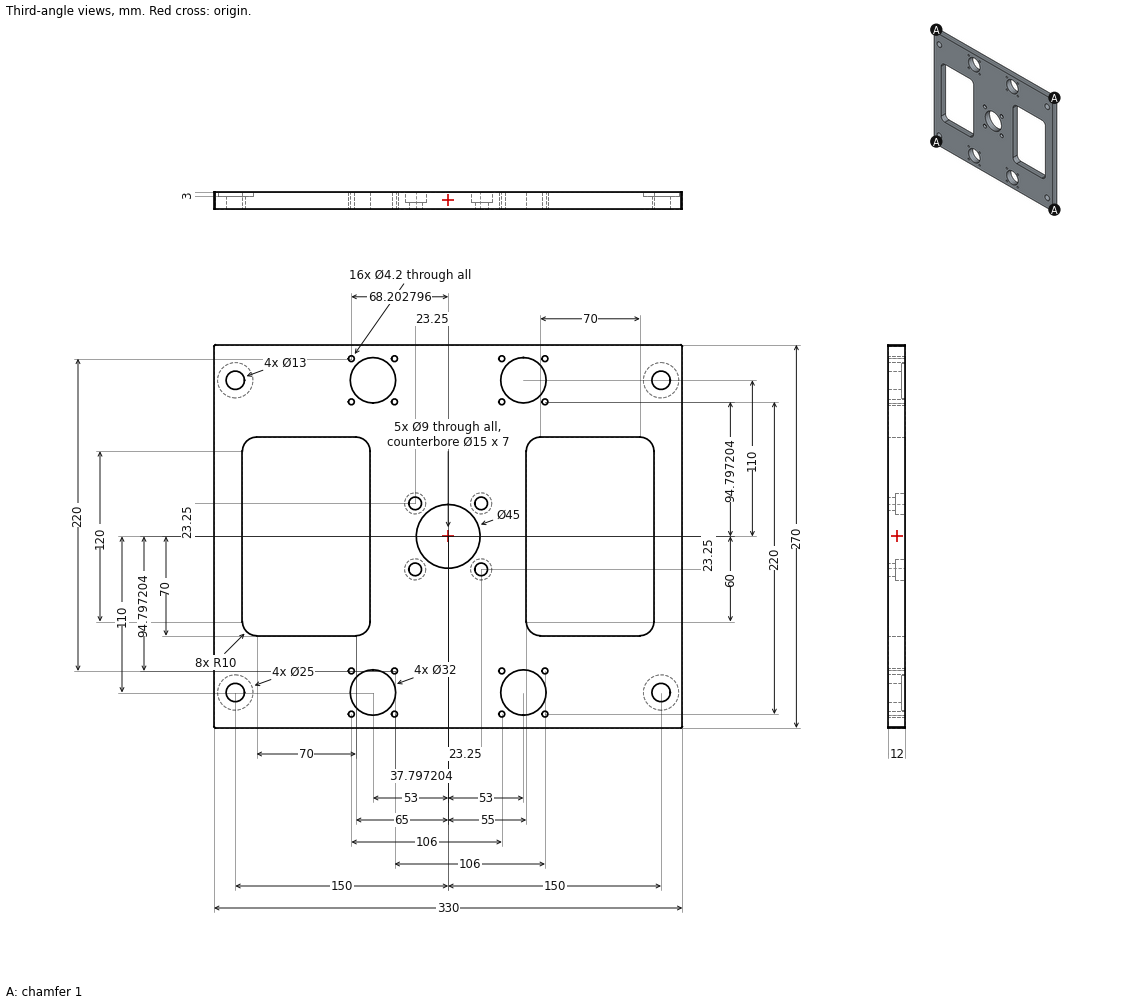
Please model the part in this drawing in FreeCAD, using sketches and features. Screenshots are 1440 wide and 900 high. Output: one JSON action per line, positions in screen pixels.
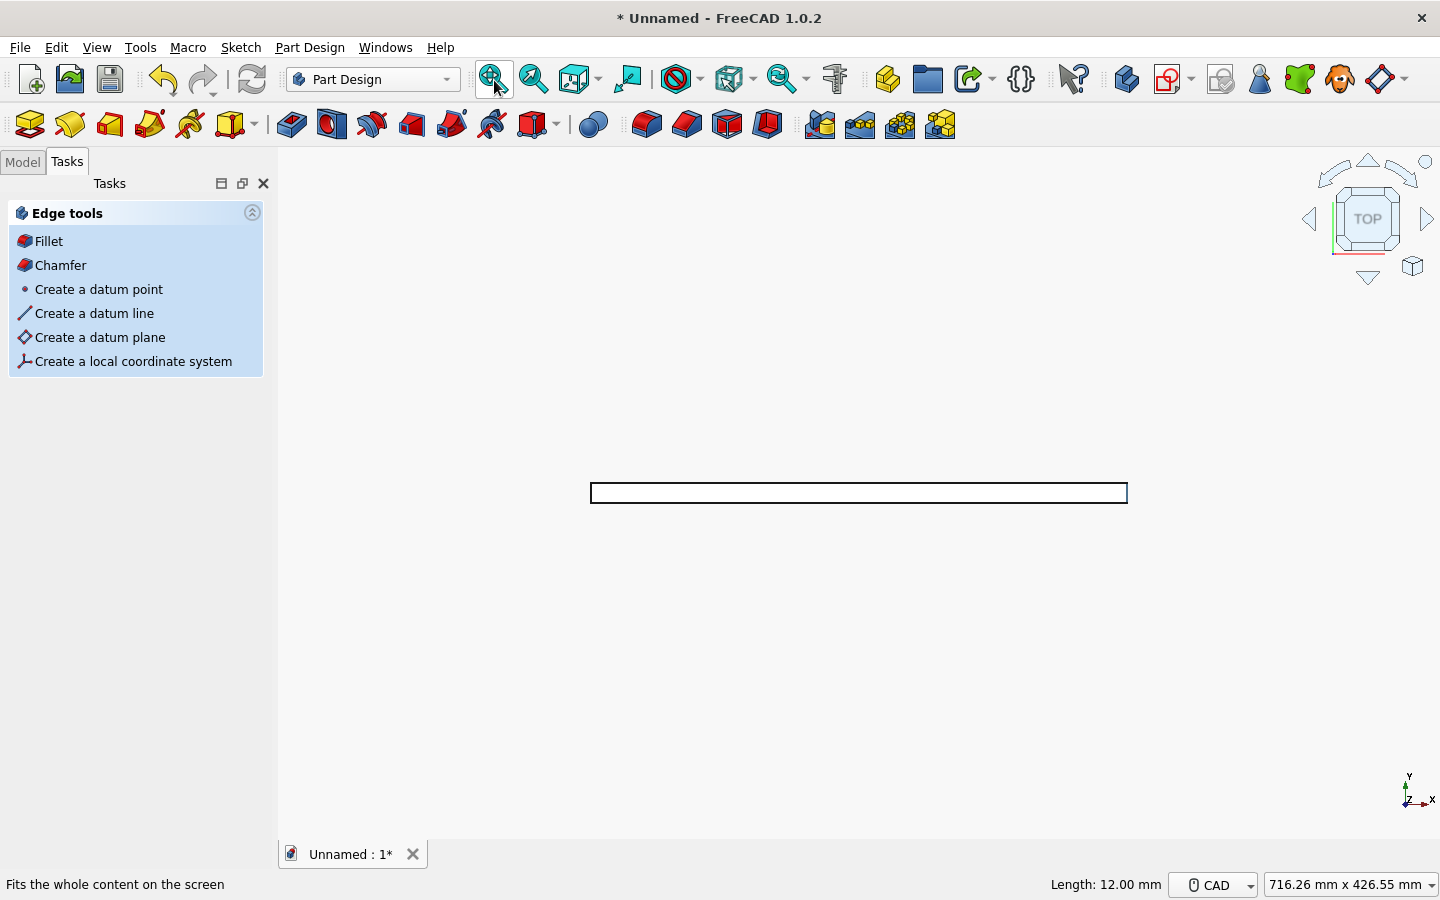
{"action": "left_click", "coordinate": [591, 492], "text": "ctrl"}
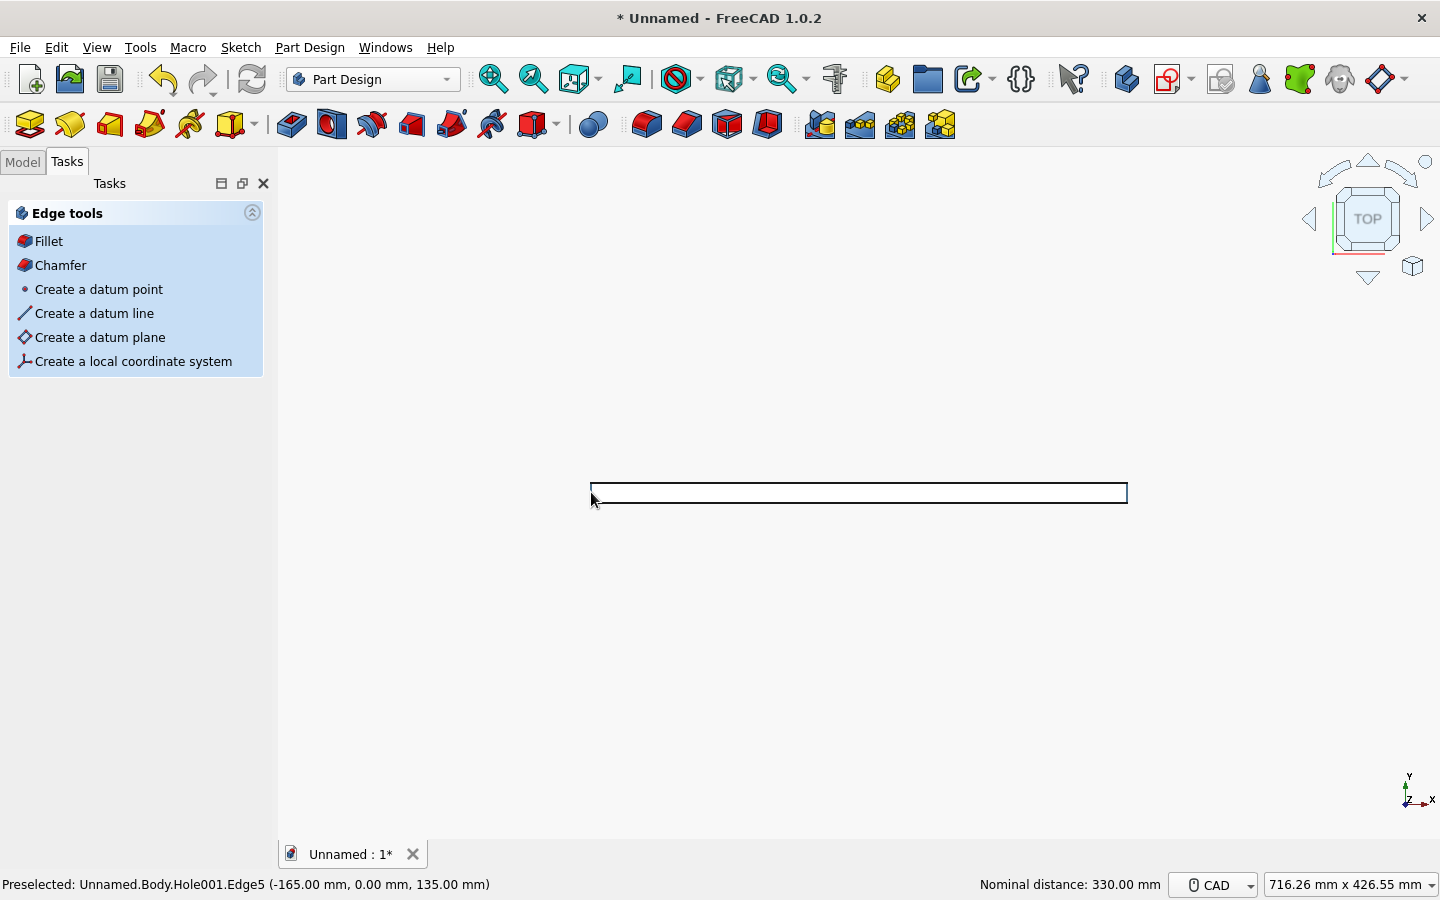
{"action": "scroll", "coordinate": [591, 492], "scroll_direction": "up", "scroll_amount": 4}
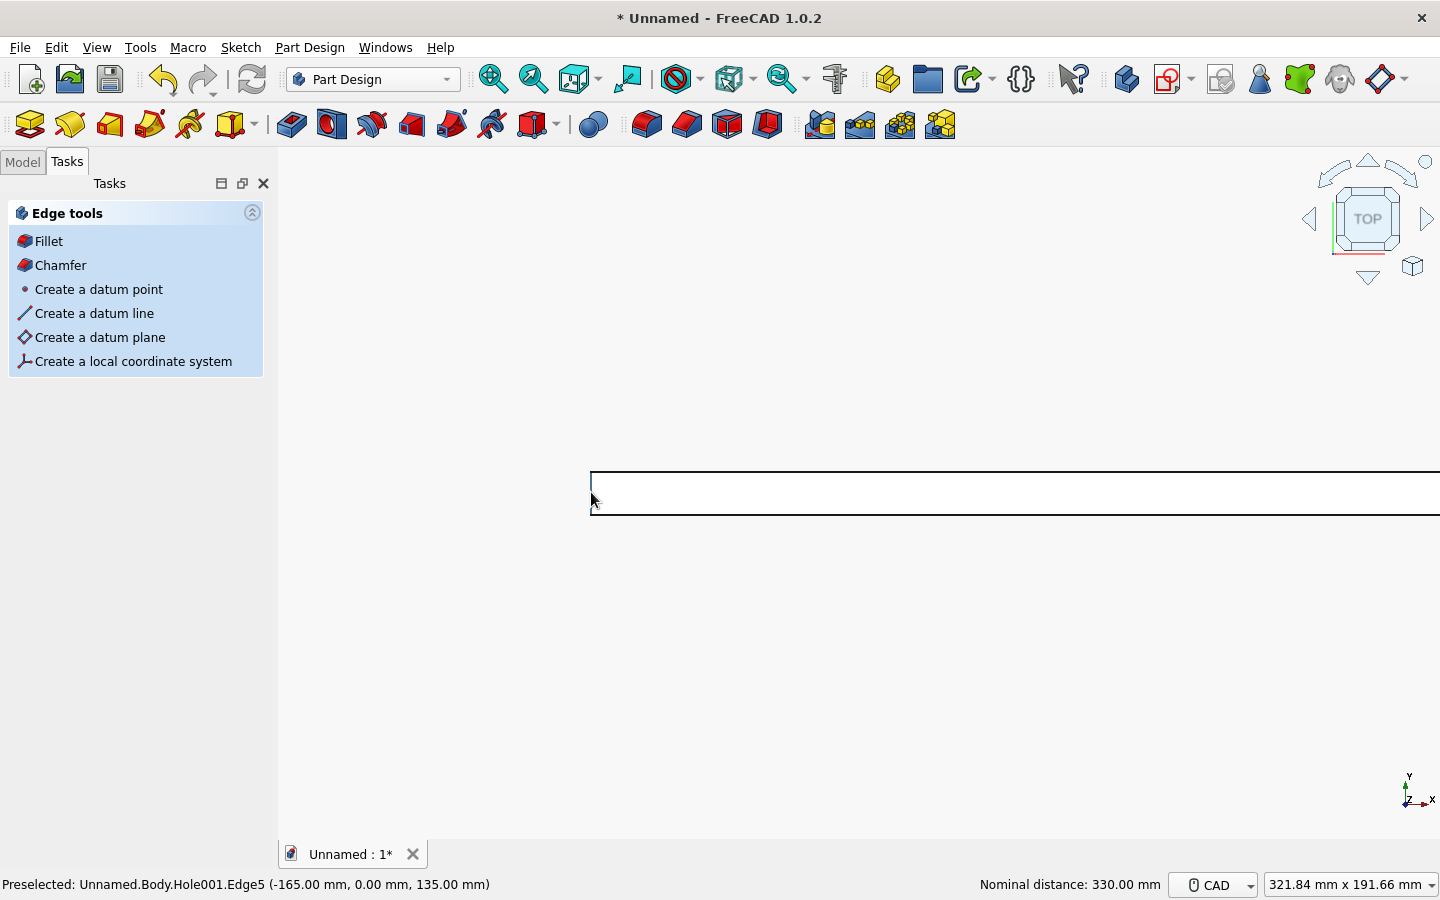
{"action": "left_click", "coordinate": [494, 80]}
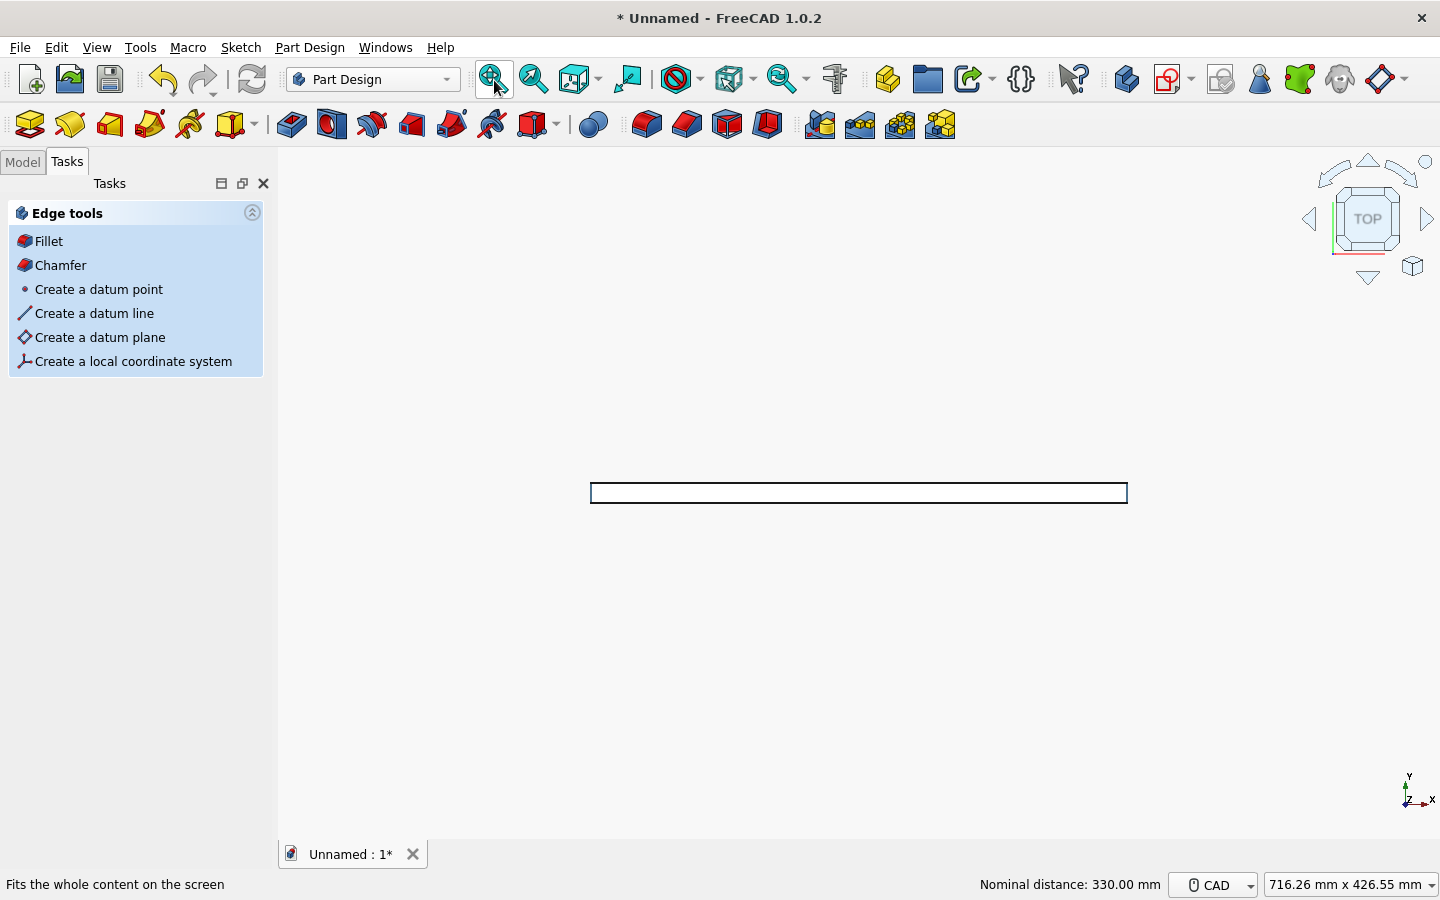
{"action": "key", "text": "1"}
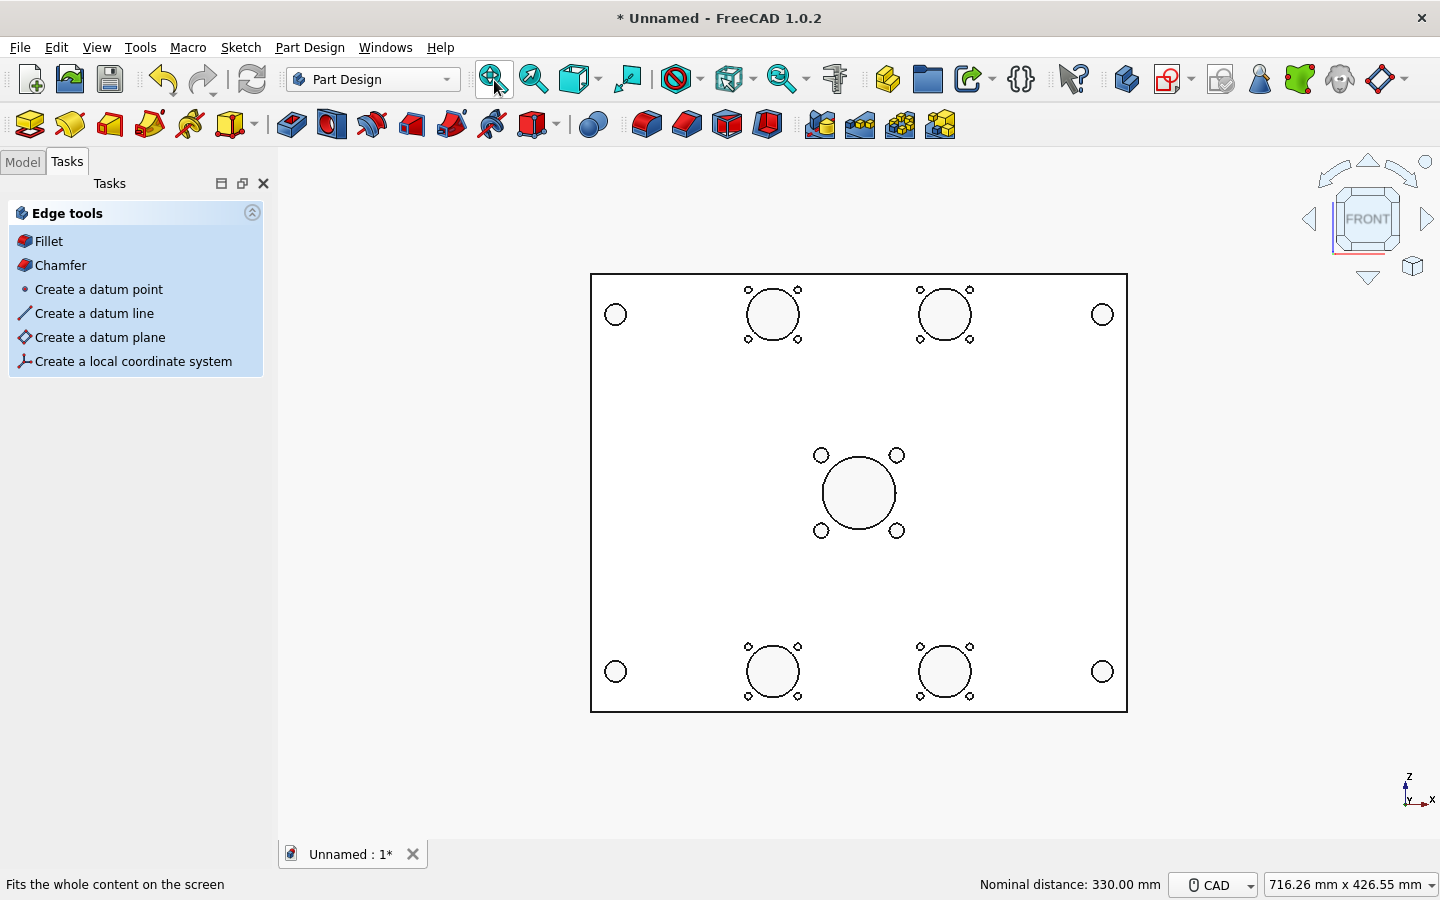
{"action": "scroll", "coordinate": [591, 711], "scroll_direction": "up", "scroll_amount": 4}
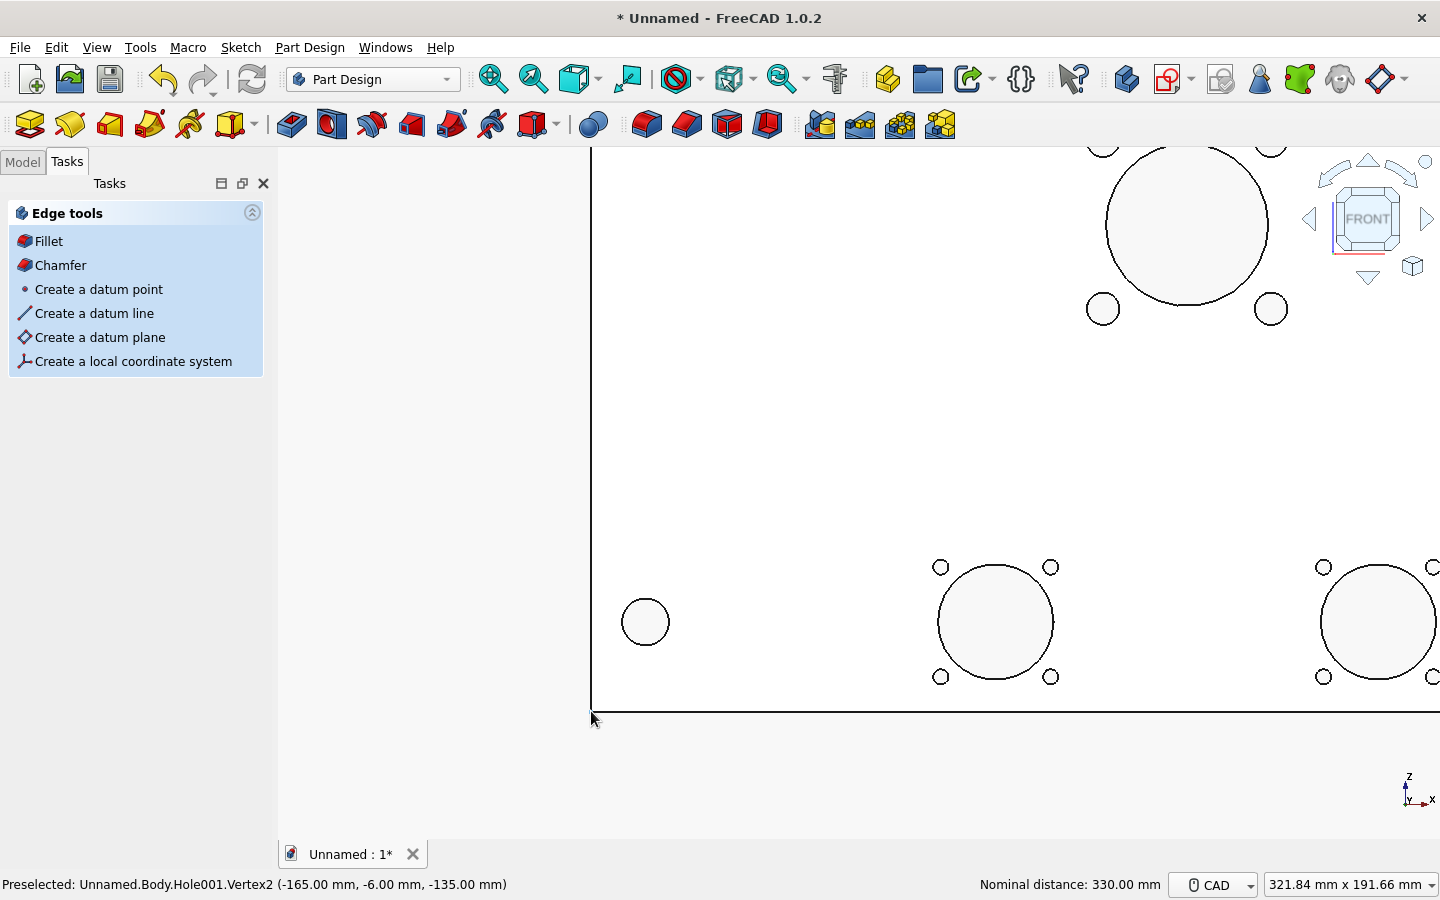
{"action": "left_click", "coordinate": [494, 80]}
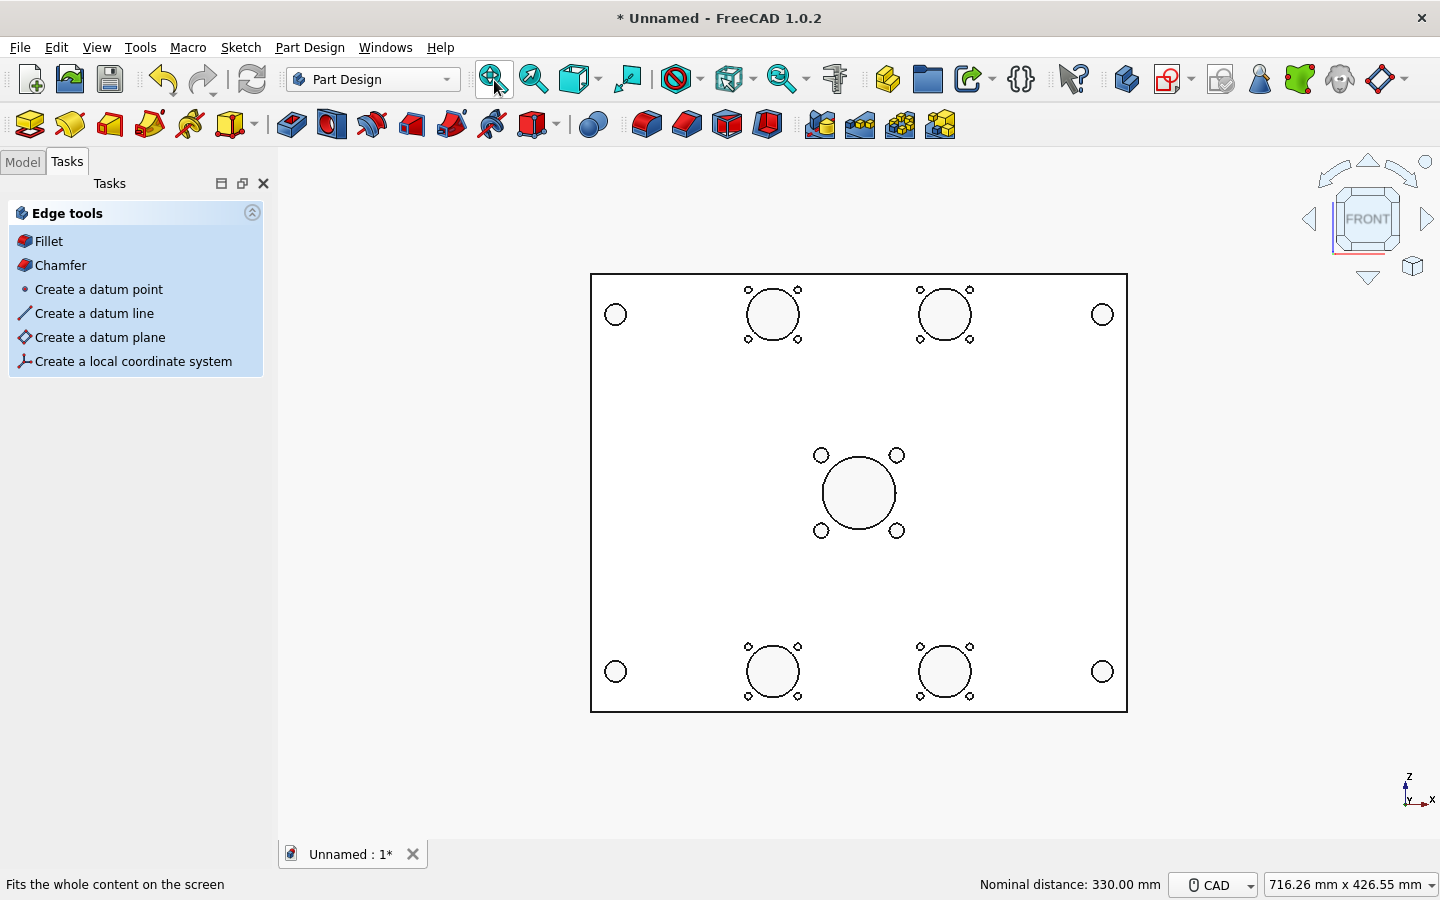
{"action": "key", "text": "3"}